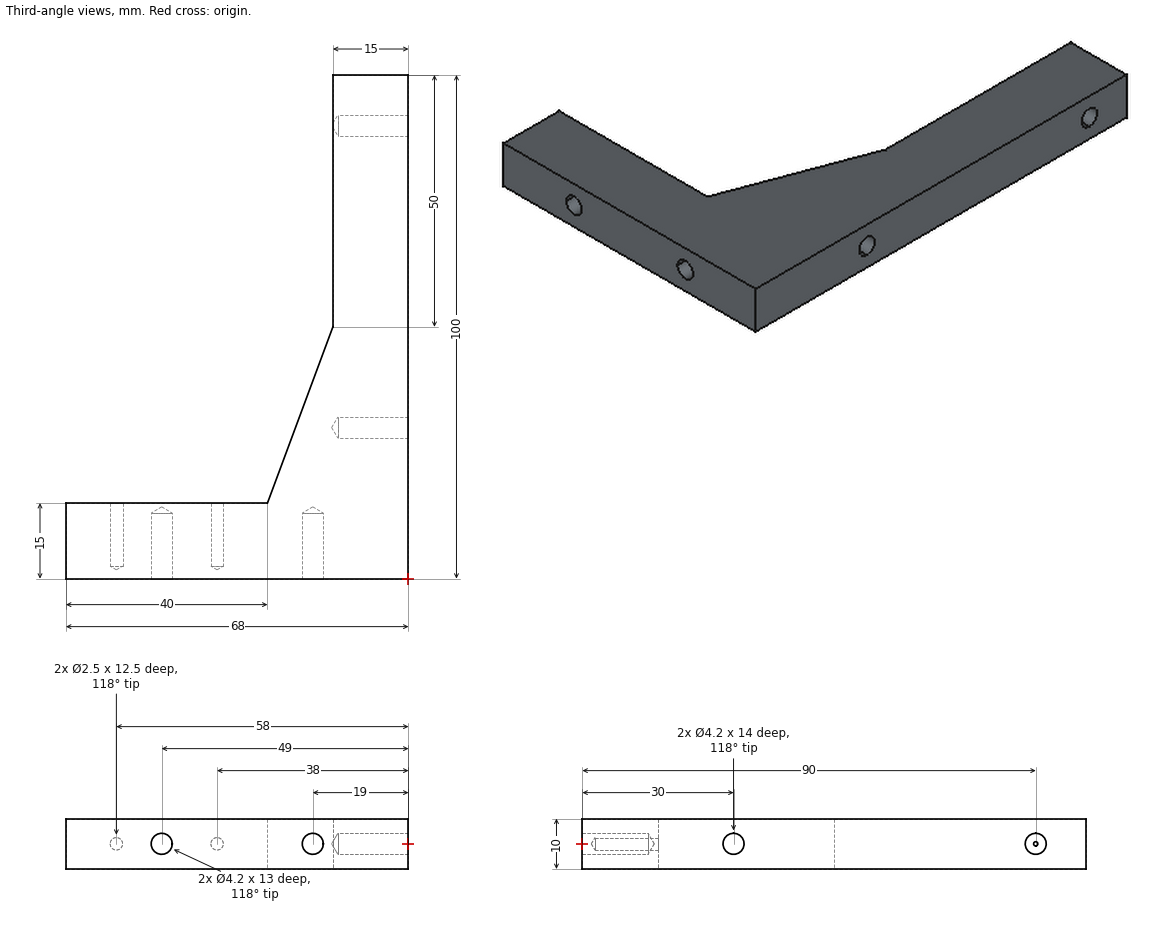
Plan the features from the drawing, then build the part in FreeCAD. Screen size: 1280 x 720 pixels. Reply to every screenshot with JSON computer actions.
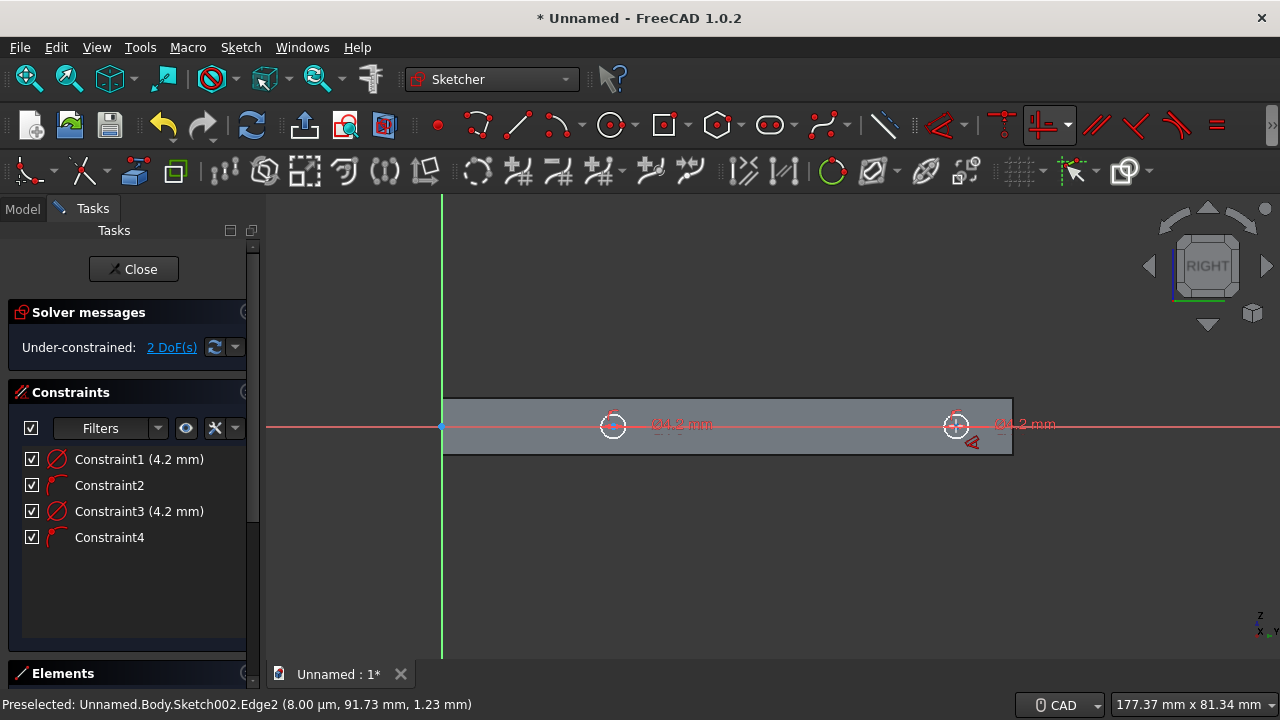
{"action": "left_click", "coordinate": [613, 426]}
{"action": "left_click", "coordinate": [527, 460]}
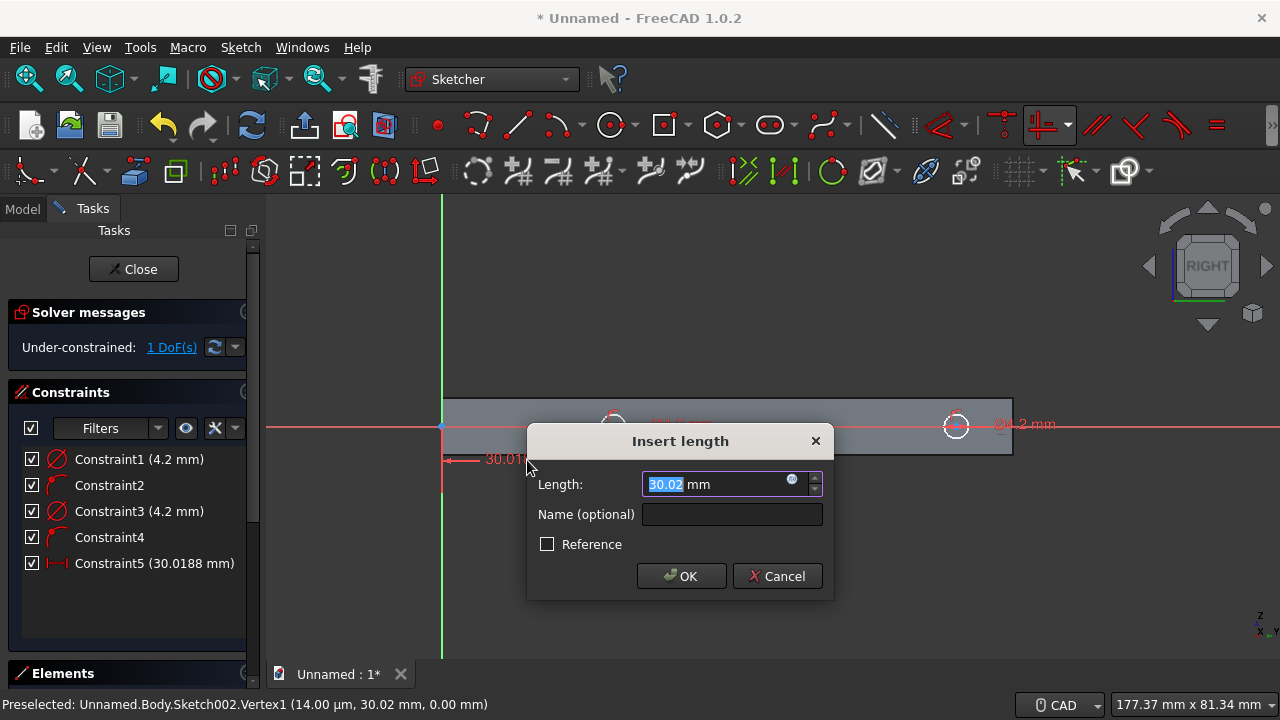
{"action": "type", "text": "30"}
{"action": "key", "text": "Return"}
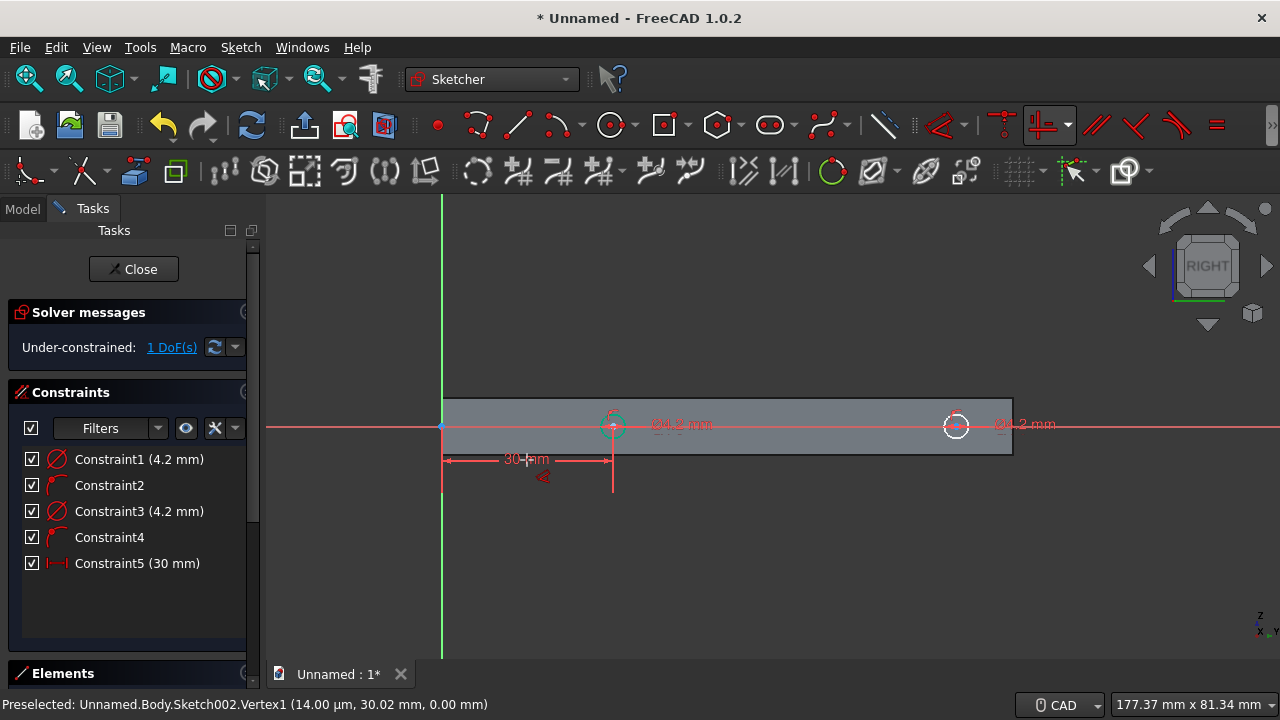
{"action": "left_click", "coordinate": [956, 426]}
{"action": "left_click", "coordinate": [699, 460]}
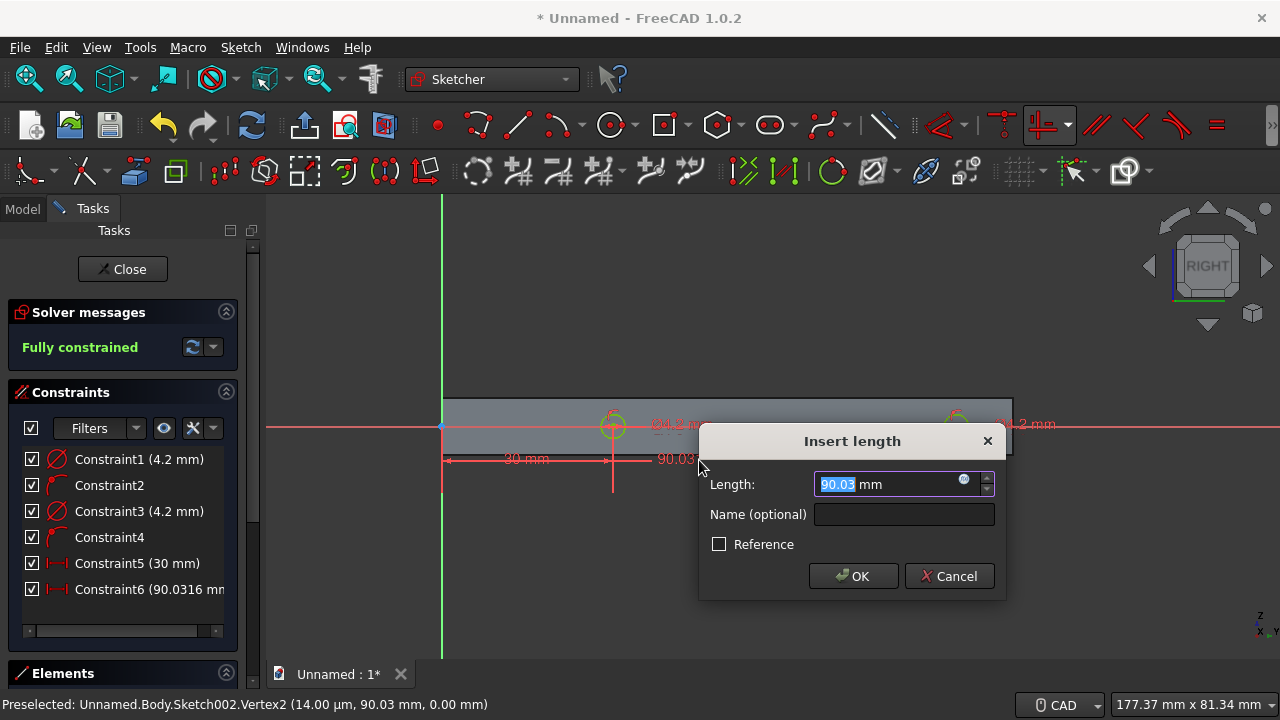
{"action": "type", "text": "90"}
{"action": "key", "text": "Return"}
{"action": "key", "text": "Escape"}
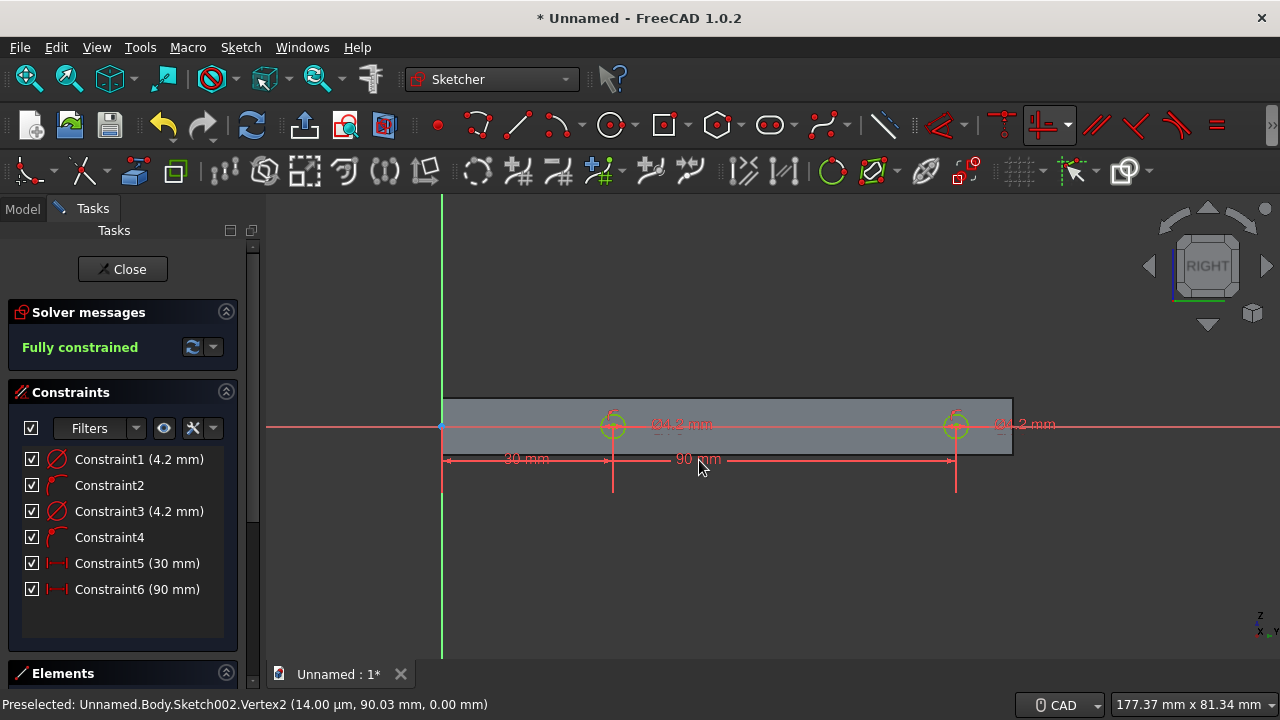
{"action": "left_click", "coordinate": [123, 269]}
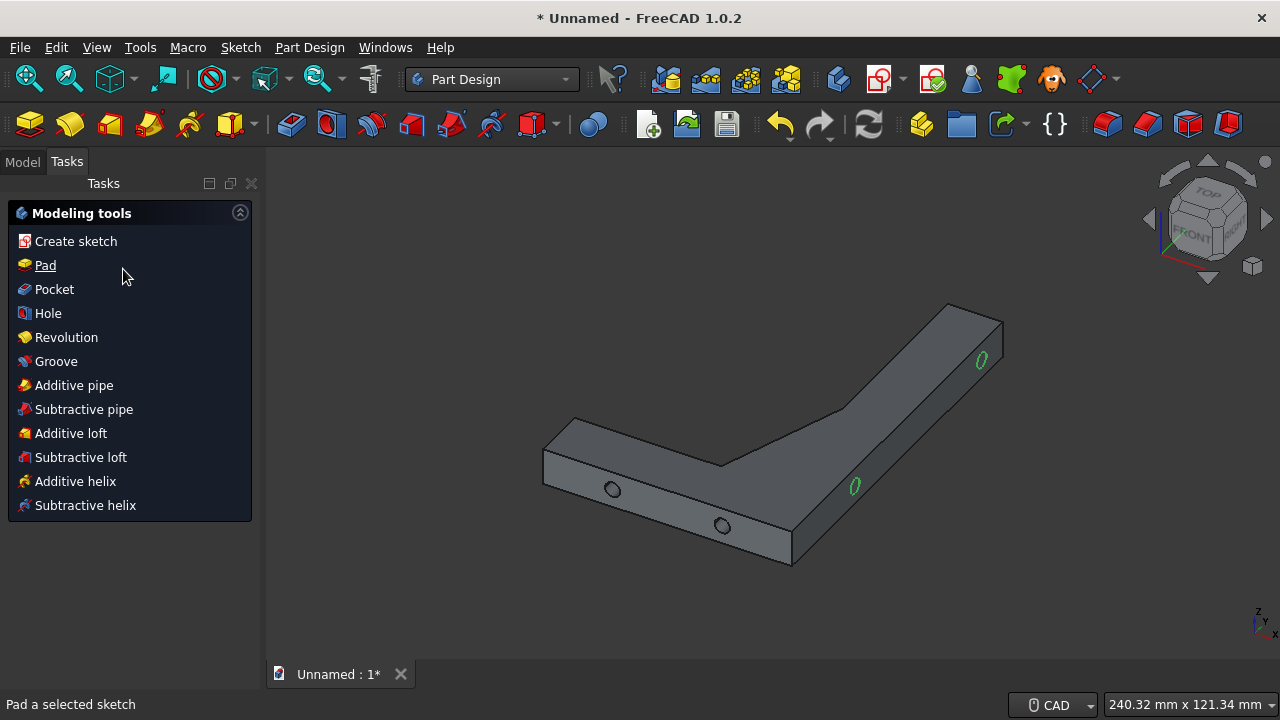
{"action": "left_click", "coordinate": [332, 124]}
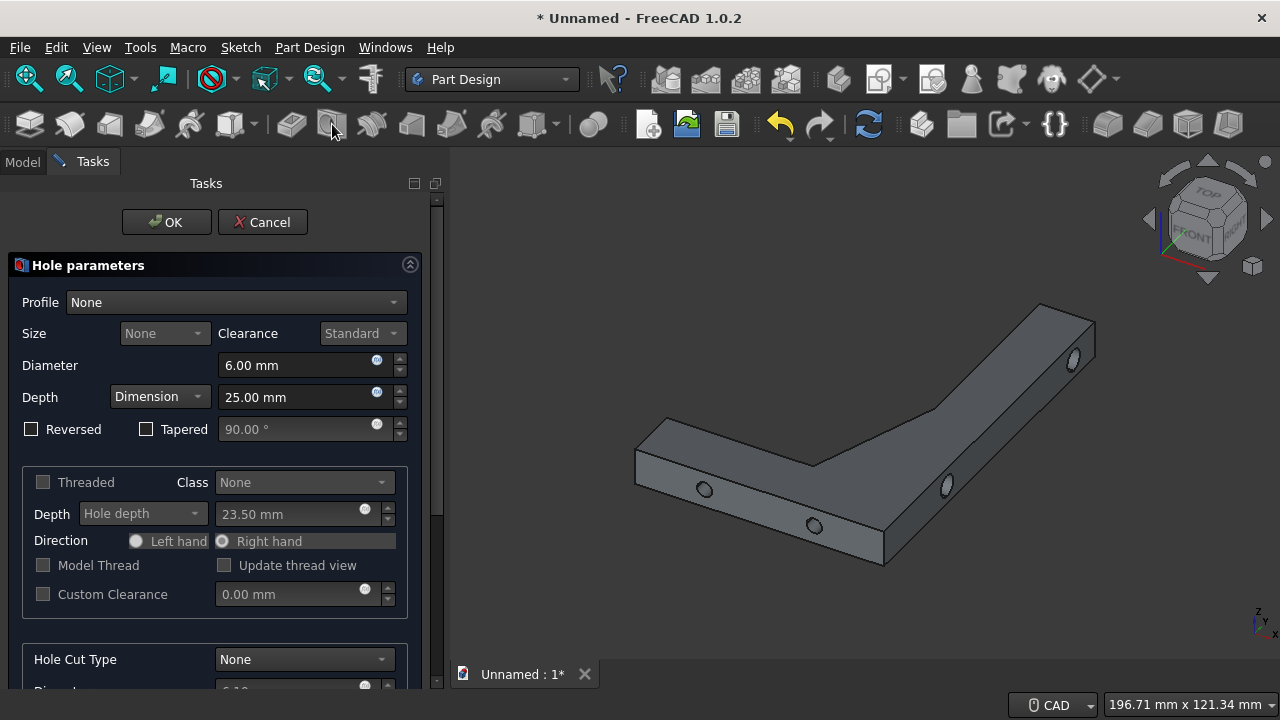
{"action": "triple_click", "coordinate": [305, 365]}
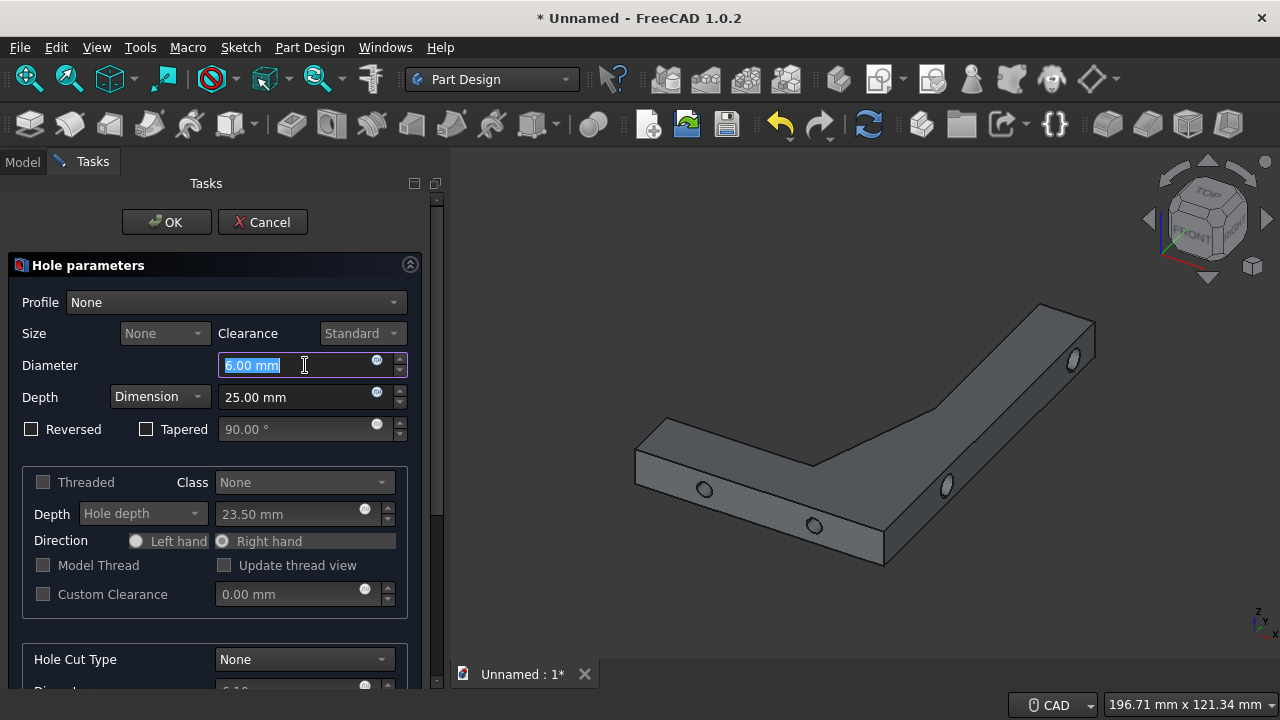
{"action": "type", "text": "4.2"}
{"action": "key", "text": "Tab"}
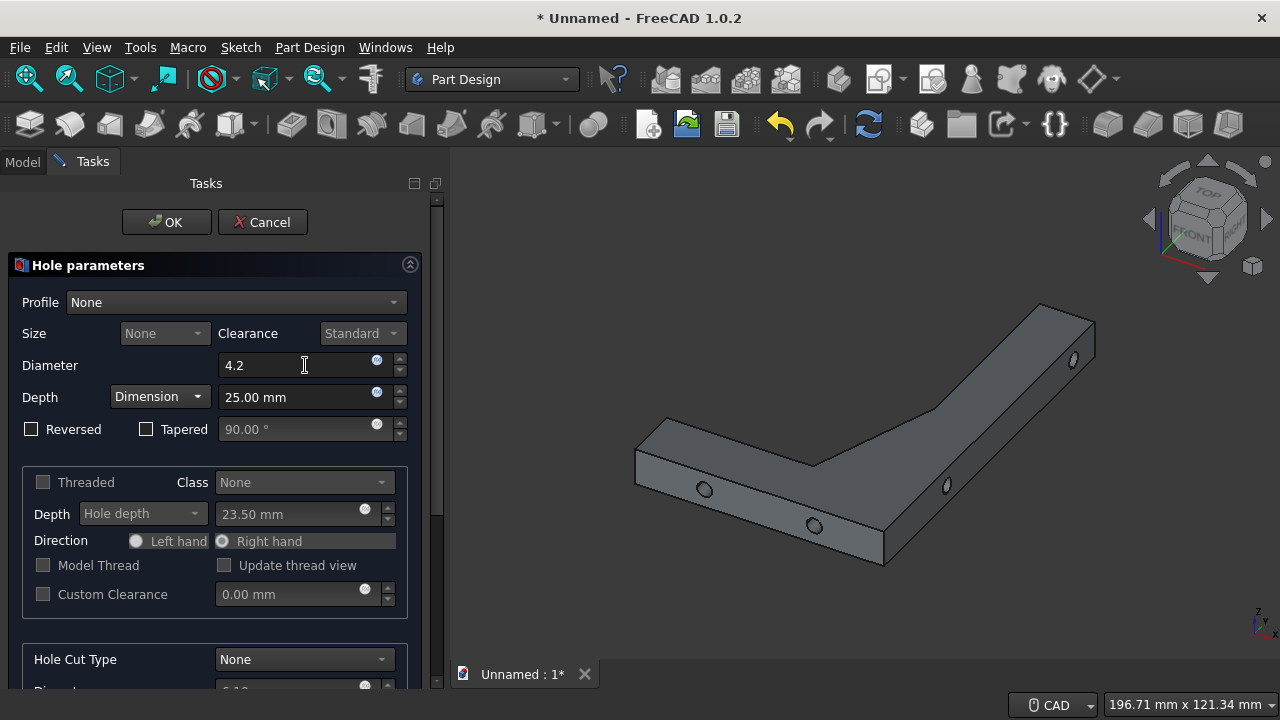
{"action": "triple_click", "coordinate": [305, 397]}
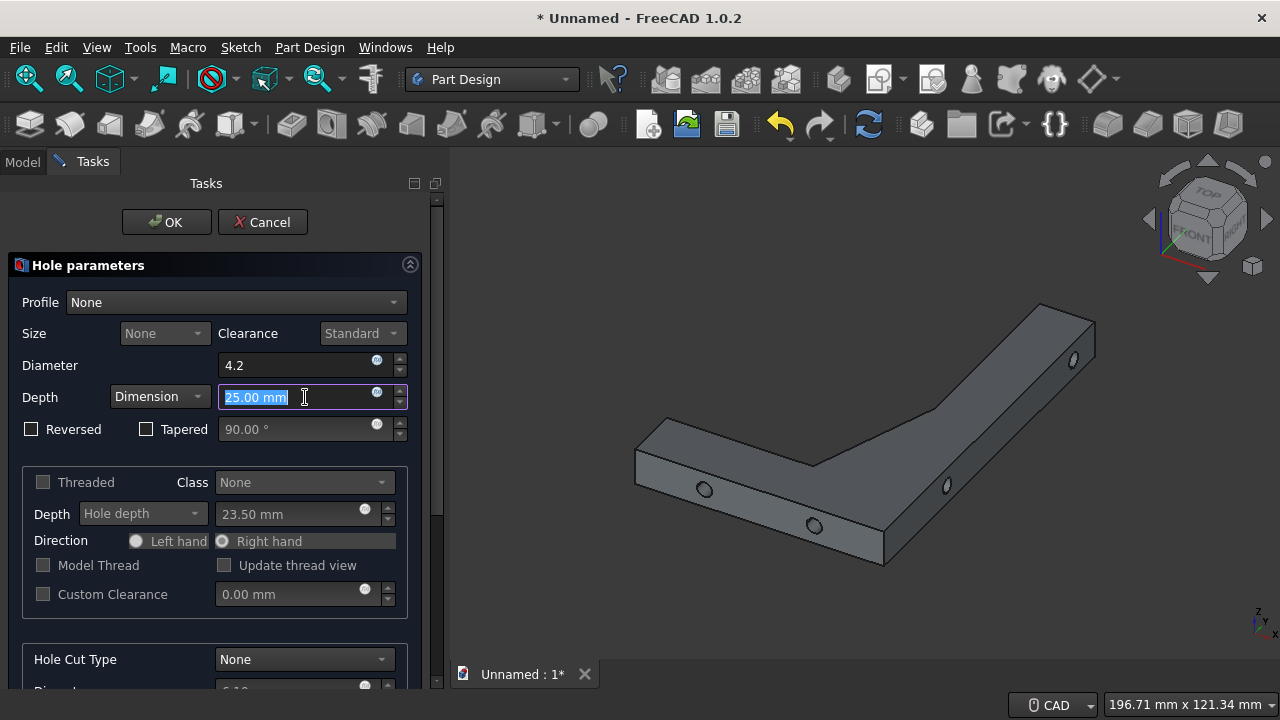
{"action": "type", "text": "14"}
{"action": "key", "text": "Tab"}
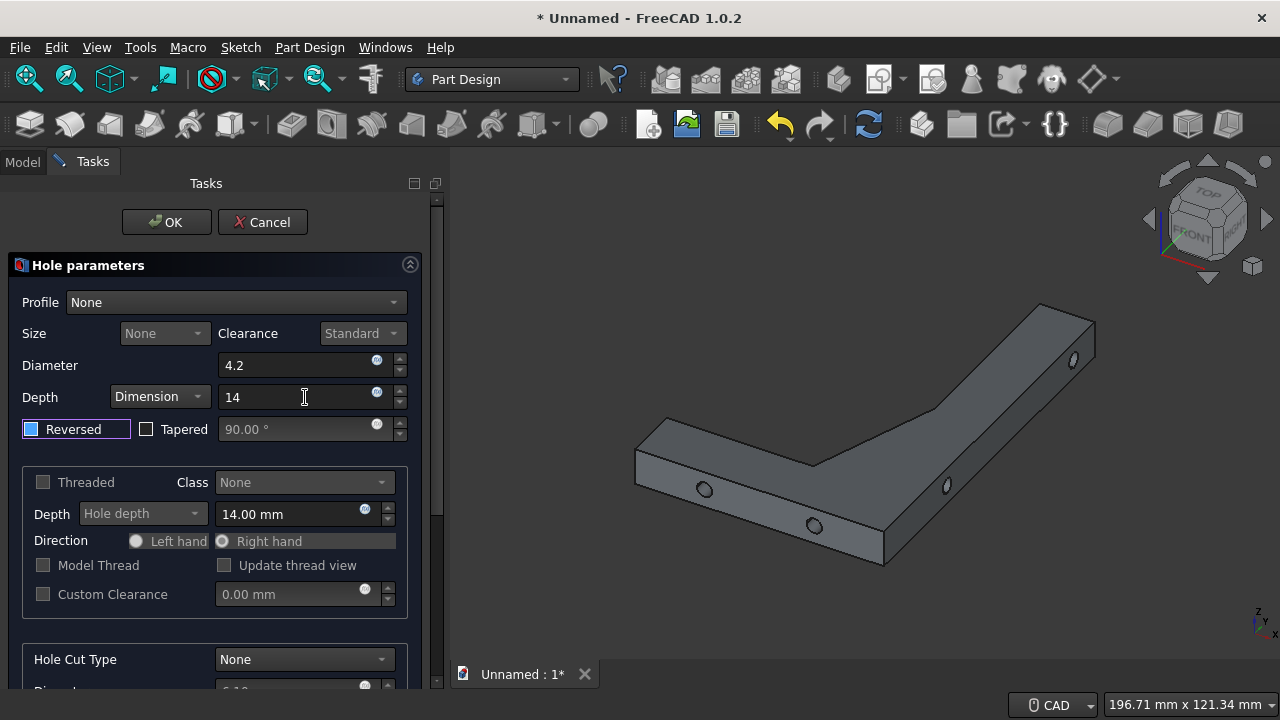
{"action": "left_click", "coordinate": [167, 222]}